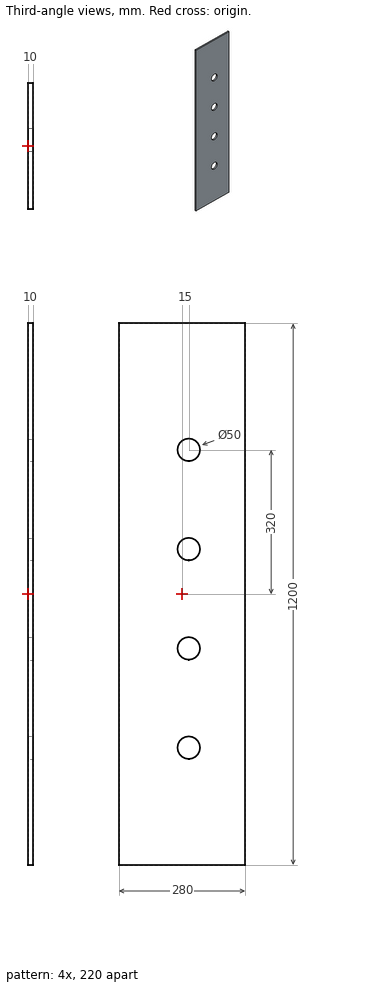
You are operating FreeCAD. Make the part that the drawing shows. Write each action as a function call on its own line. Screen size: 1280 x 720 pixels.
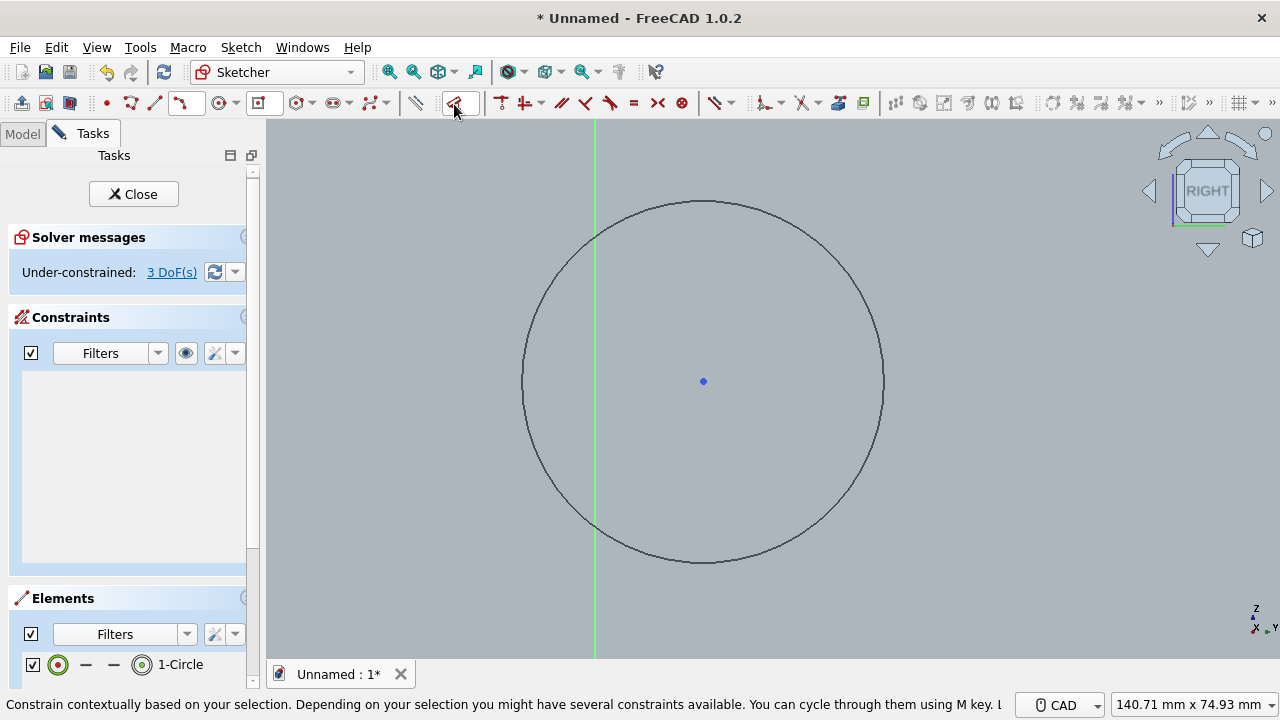
click(831, 254)
click(854, 231)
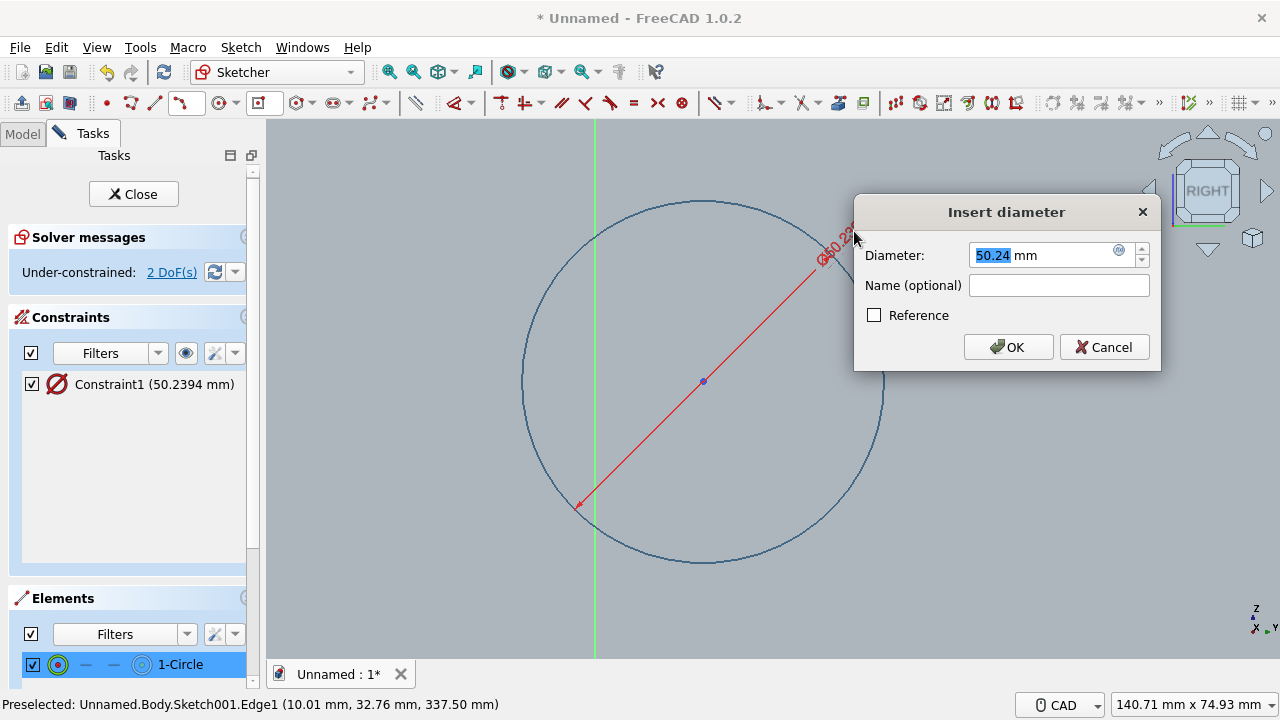
text(50)
key(Return)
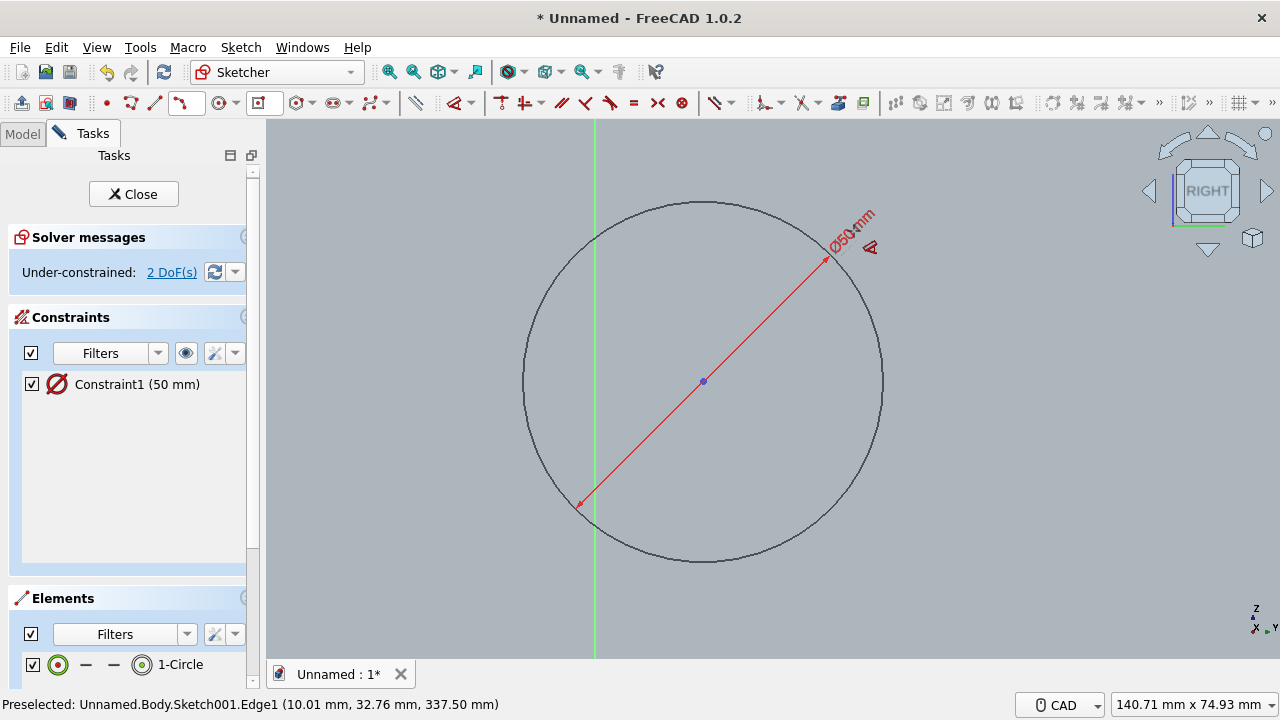
click(703, 382)
click(649, 348)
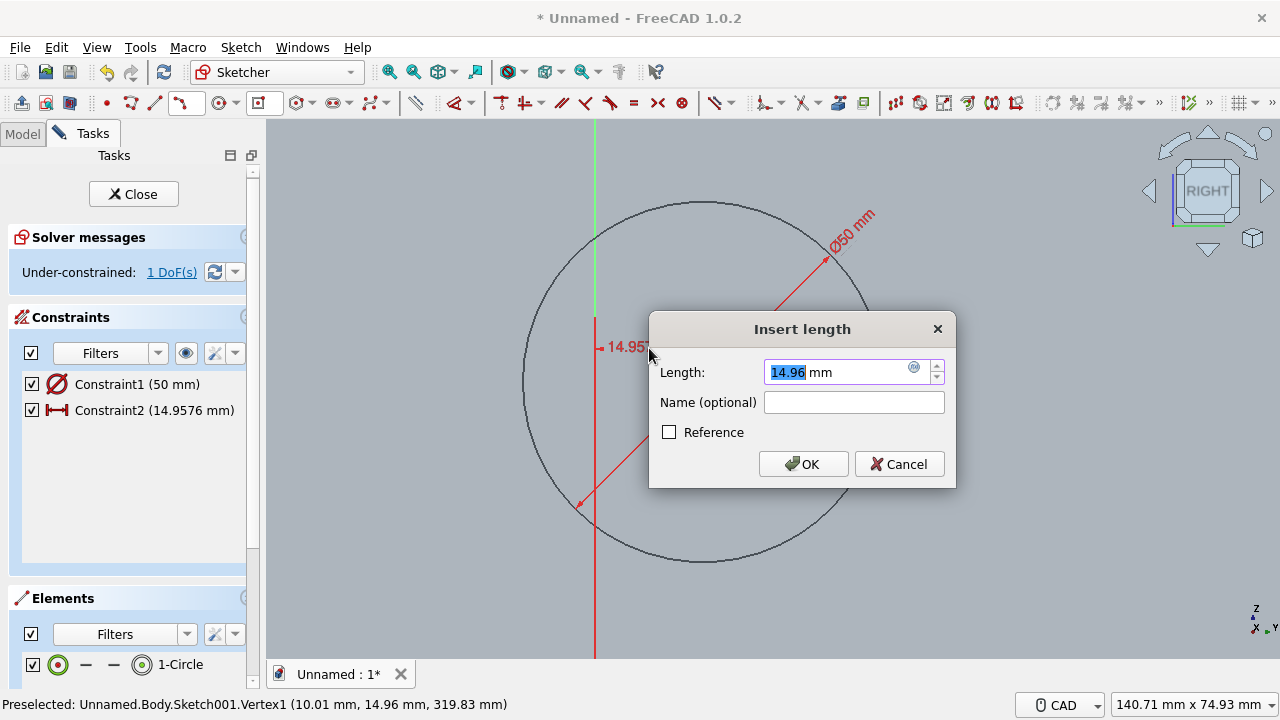
text(15)
key(Return)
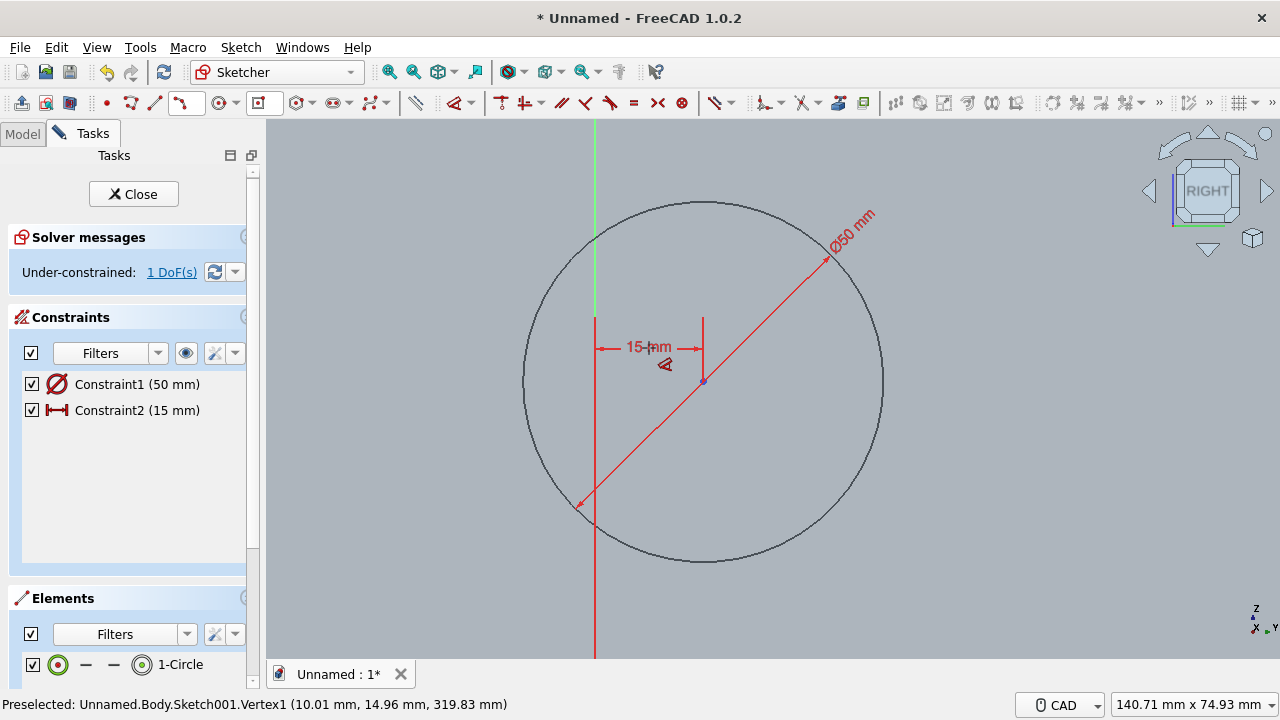
click(703, 382)
click(561, 449)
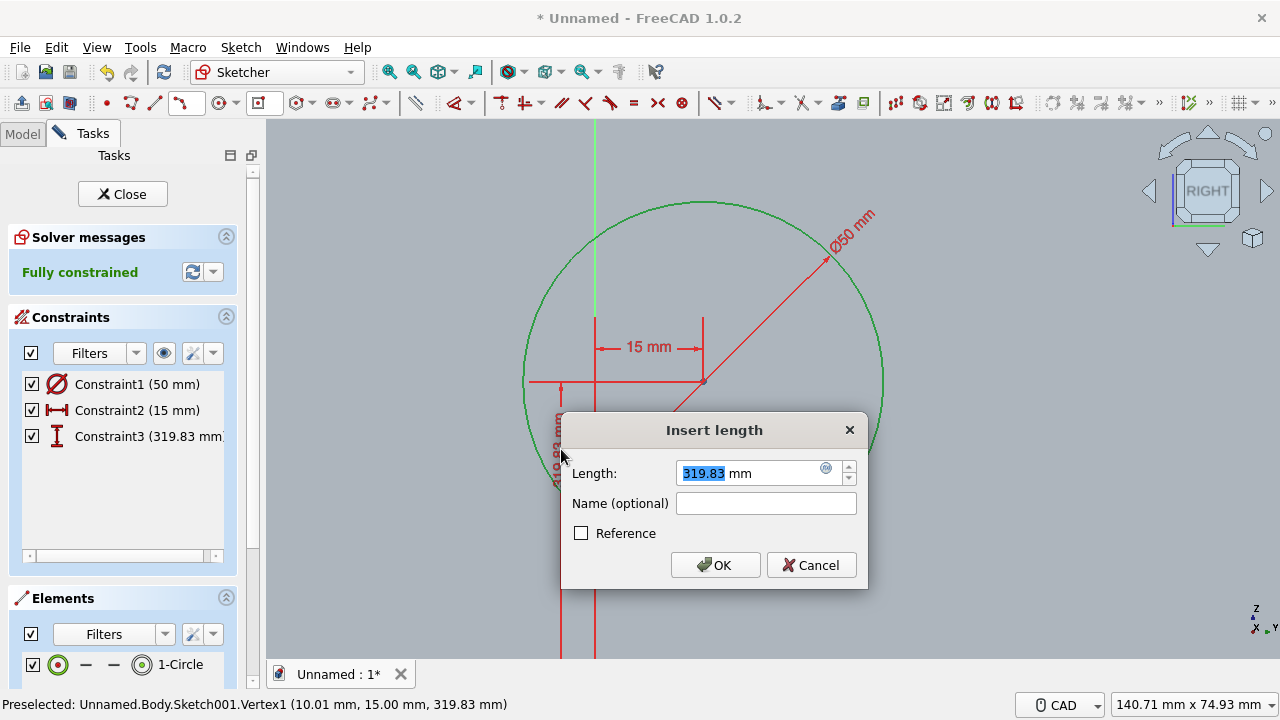
text(320)
key(Return)
key(Escape)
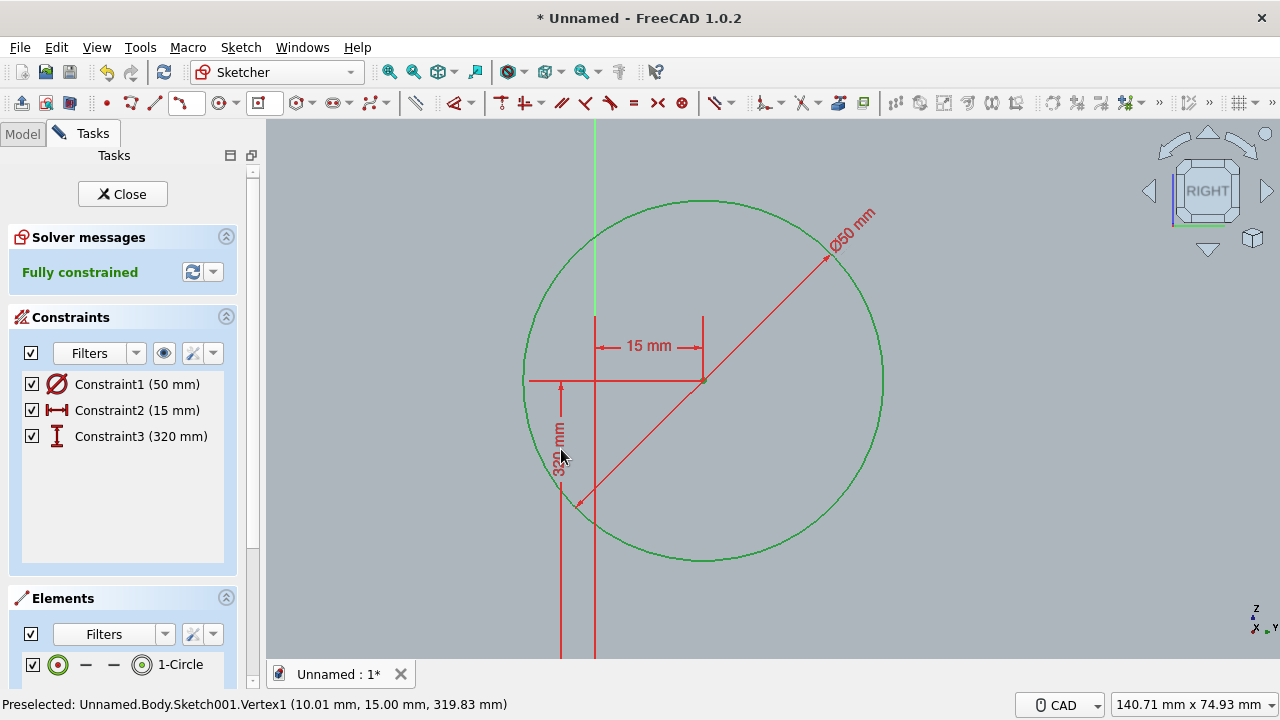
click(123, 194)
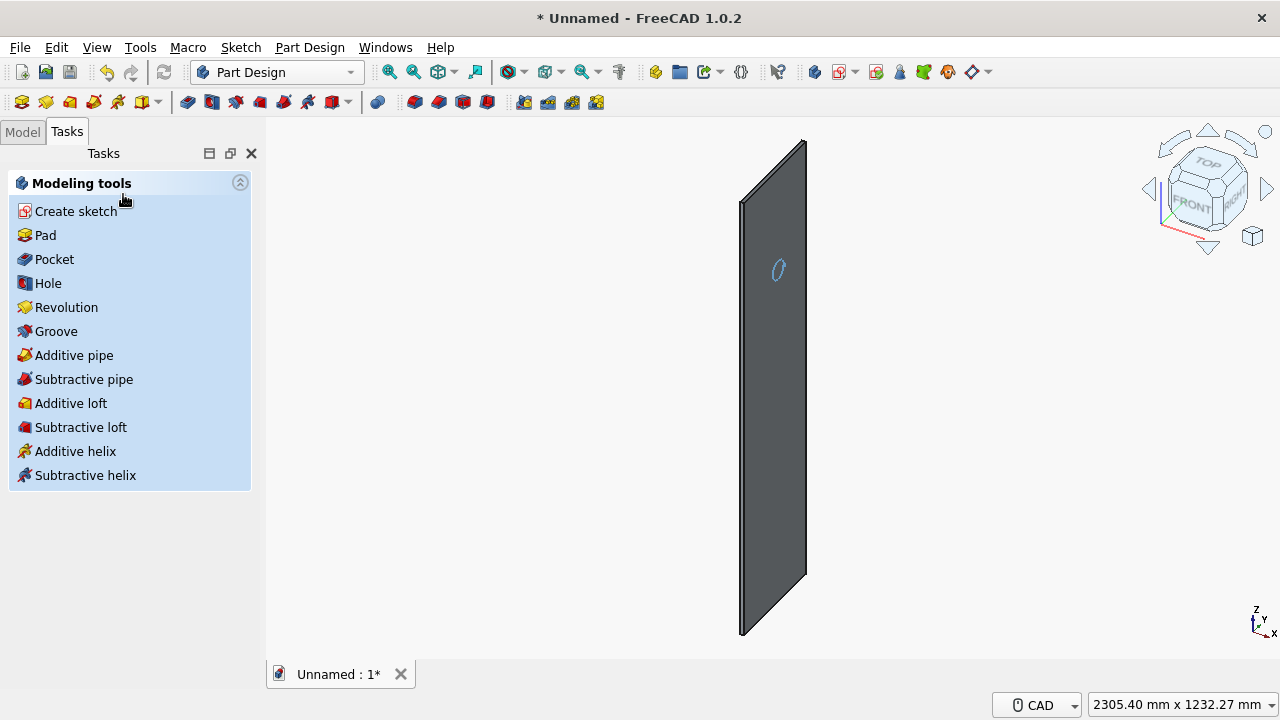
click(188, 102)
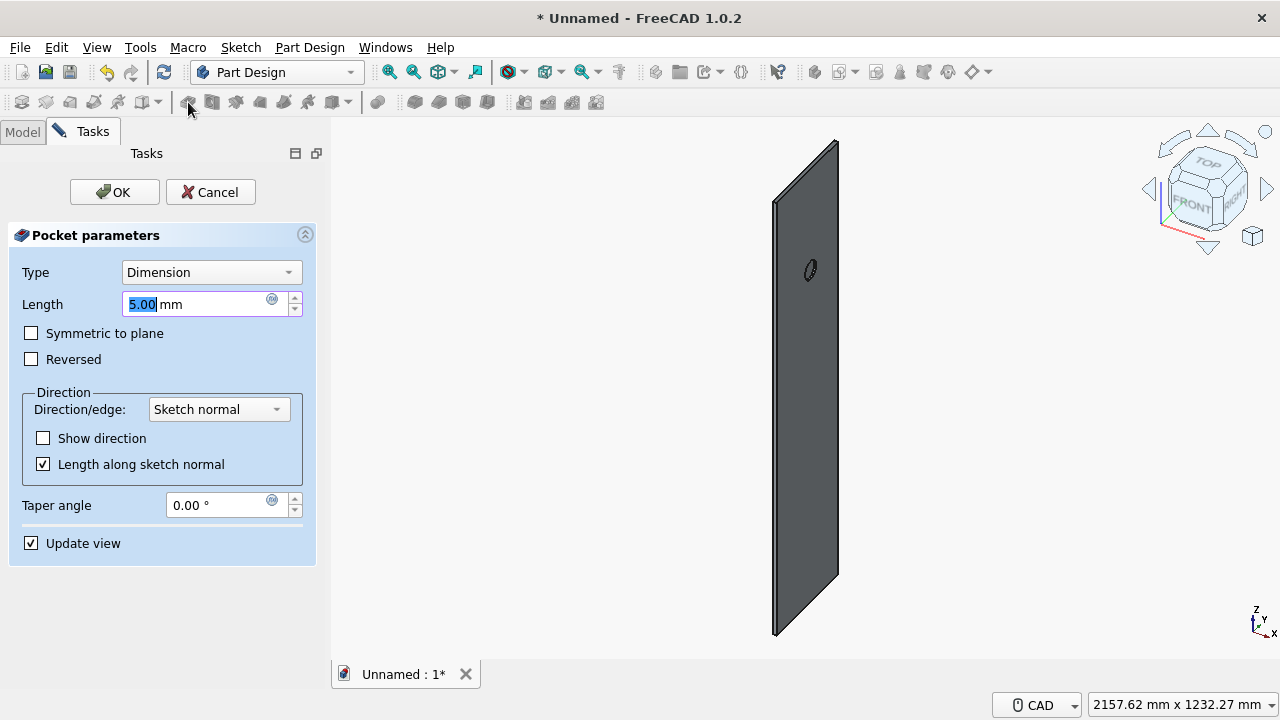
text(10)
key(Tab)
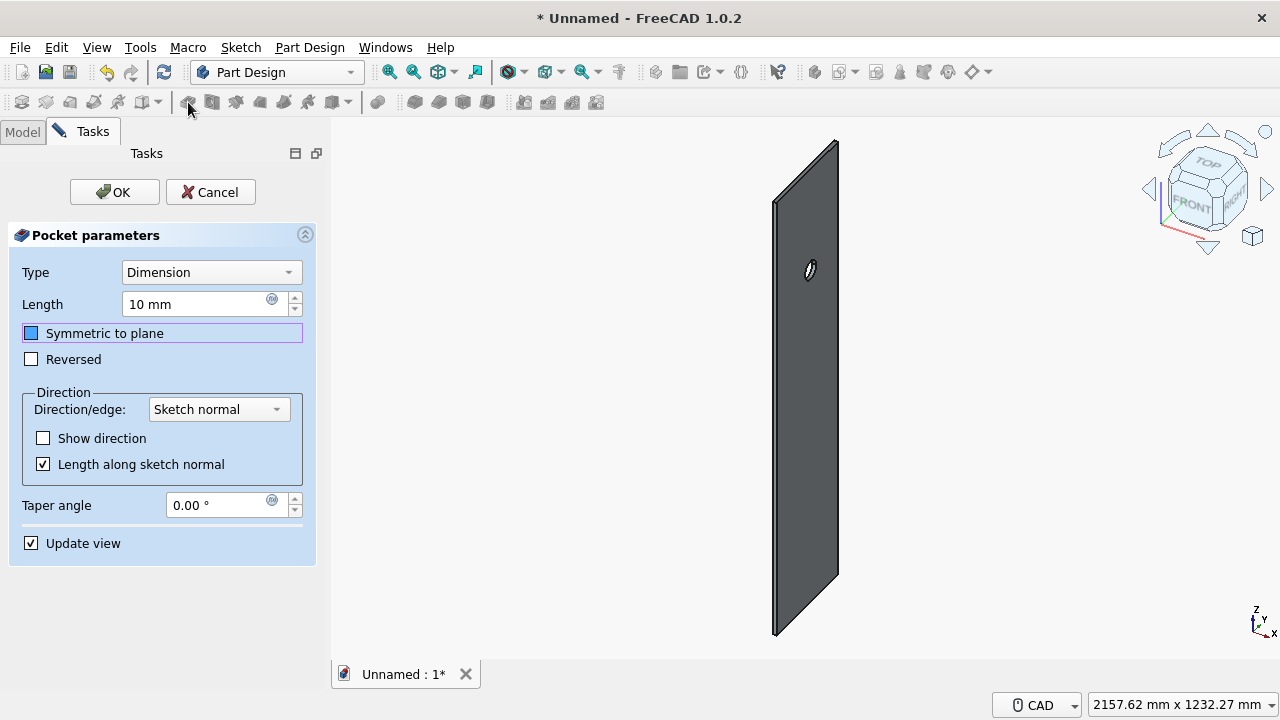
click(115, 192)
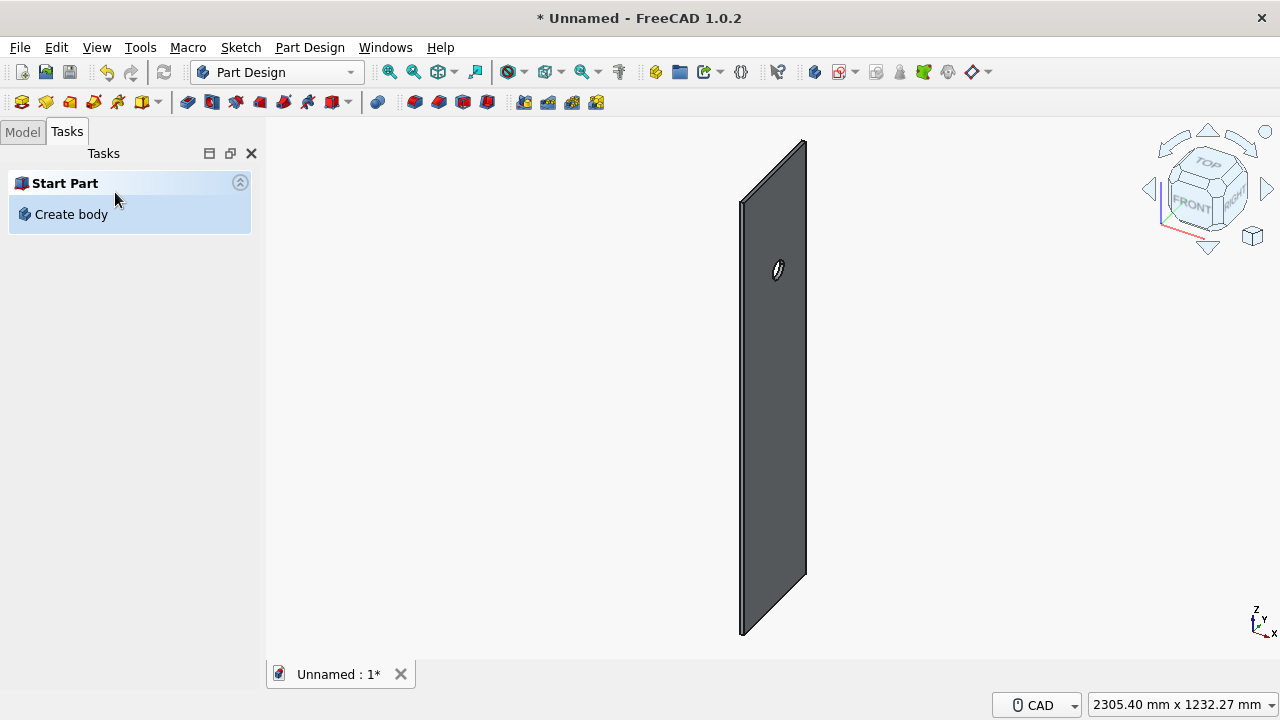
click(23, 131)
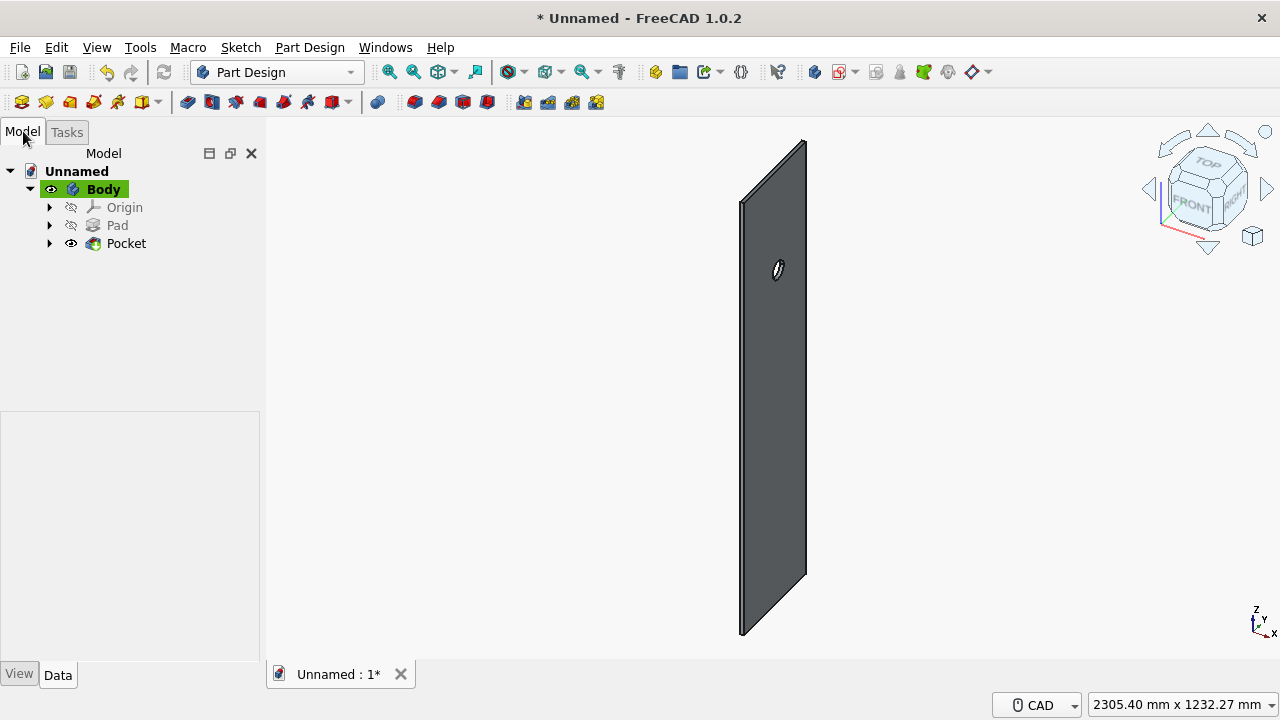
click(116, 243)